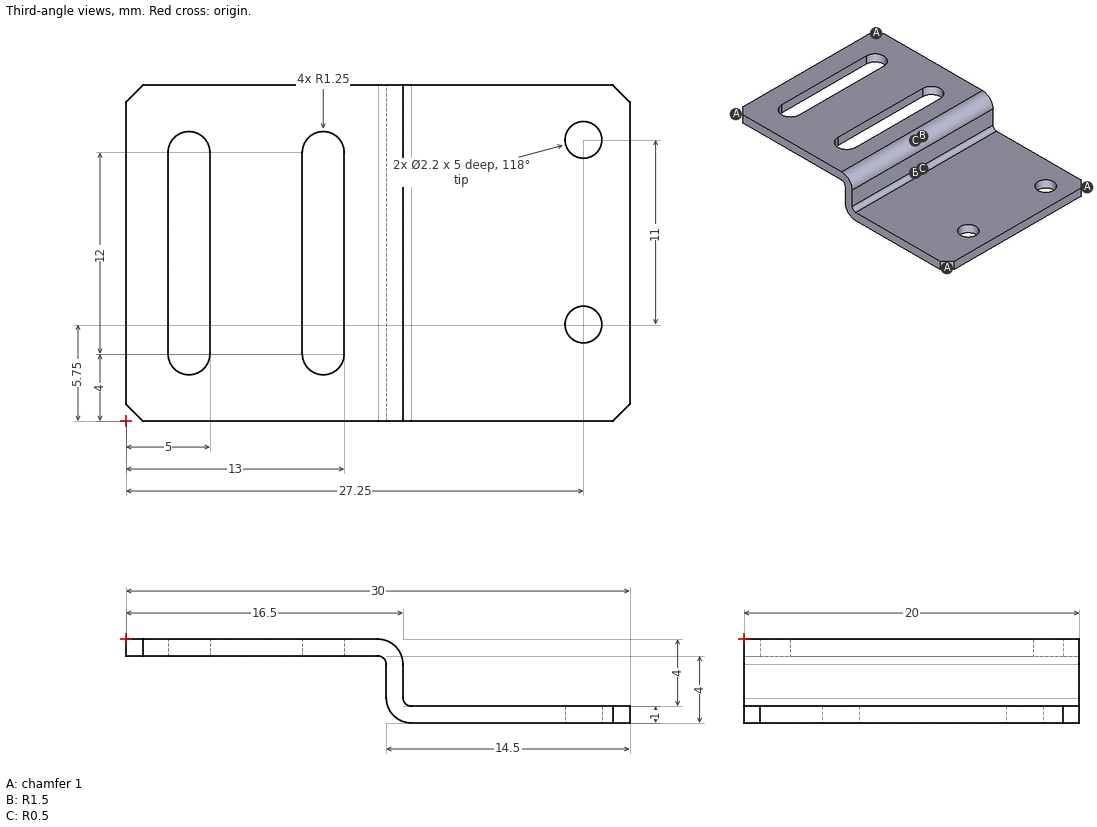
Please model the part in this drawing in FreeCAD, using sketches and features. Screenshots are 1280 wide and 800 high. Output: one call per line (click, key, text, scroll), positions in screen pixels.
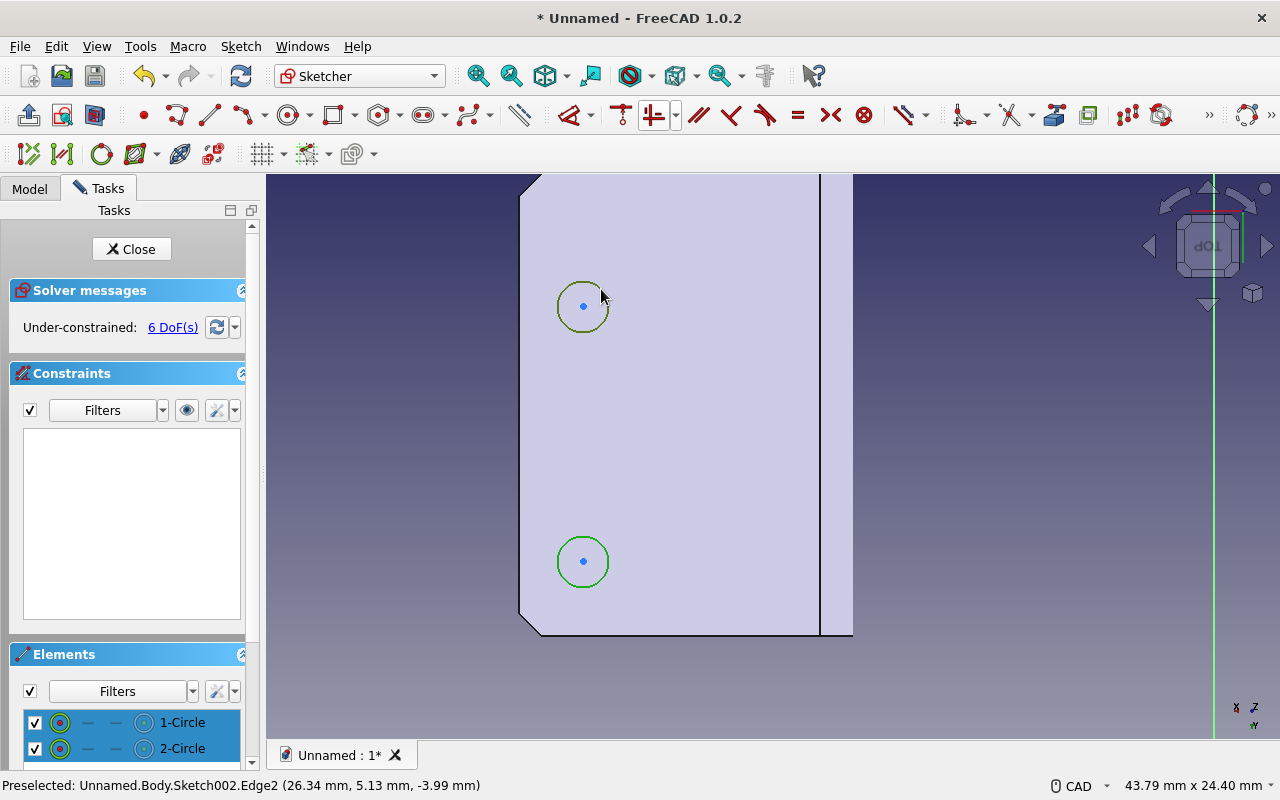
click(798, 116)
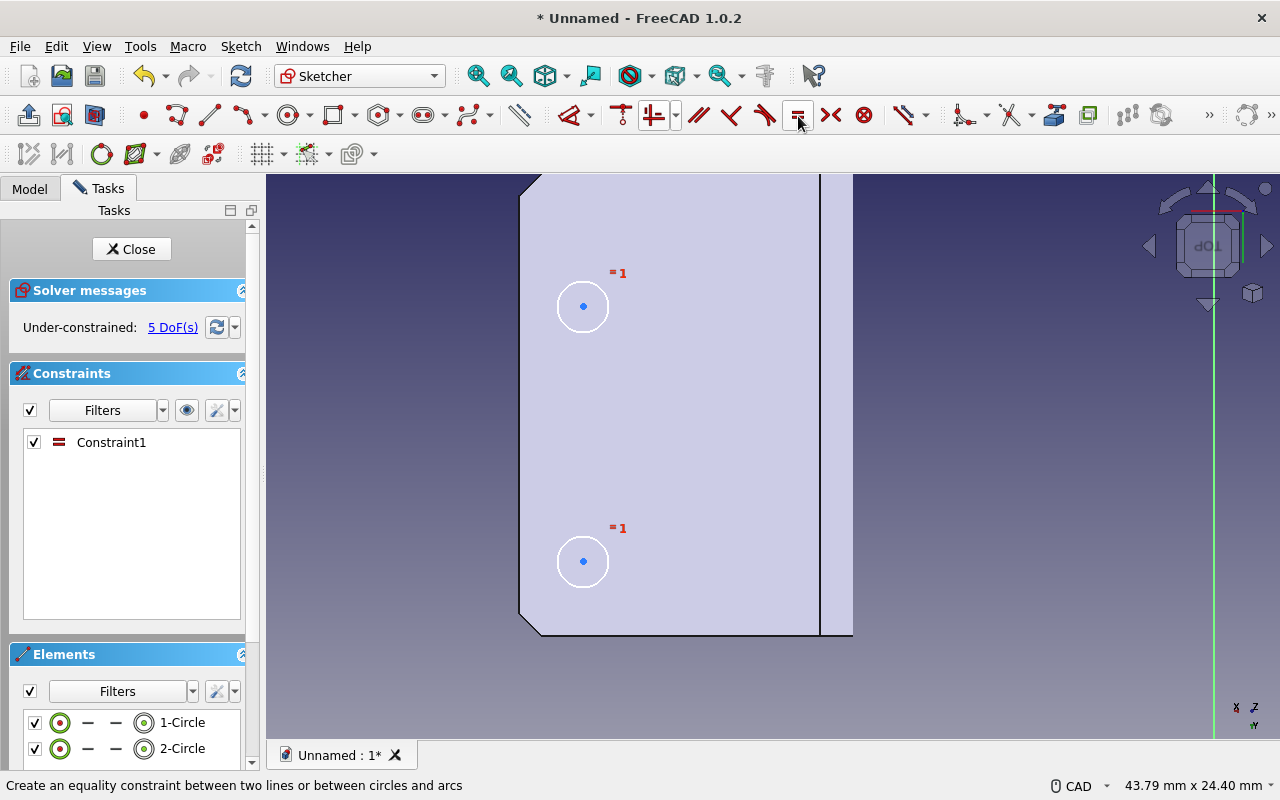
click(583, 562)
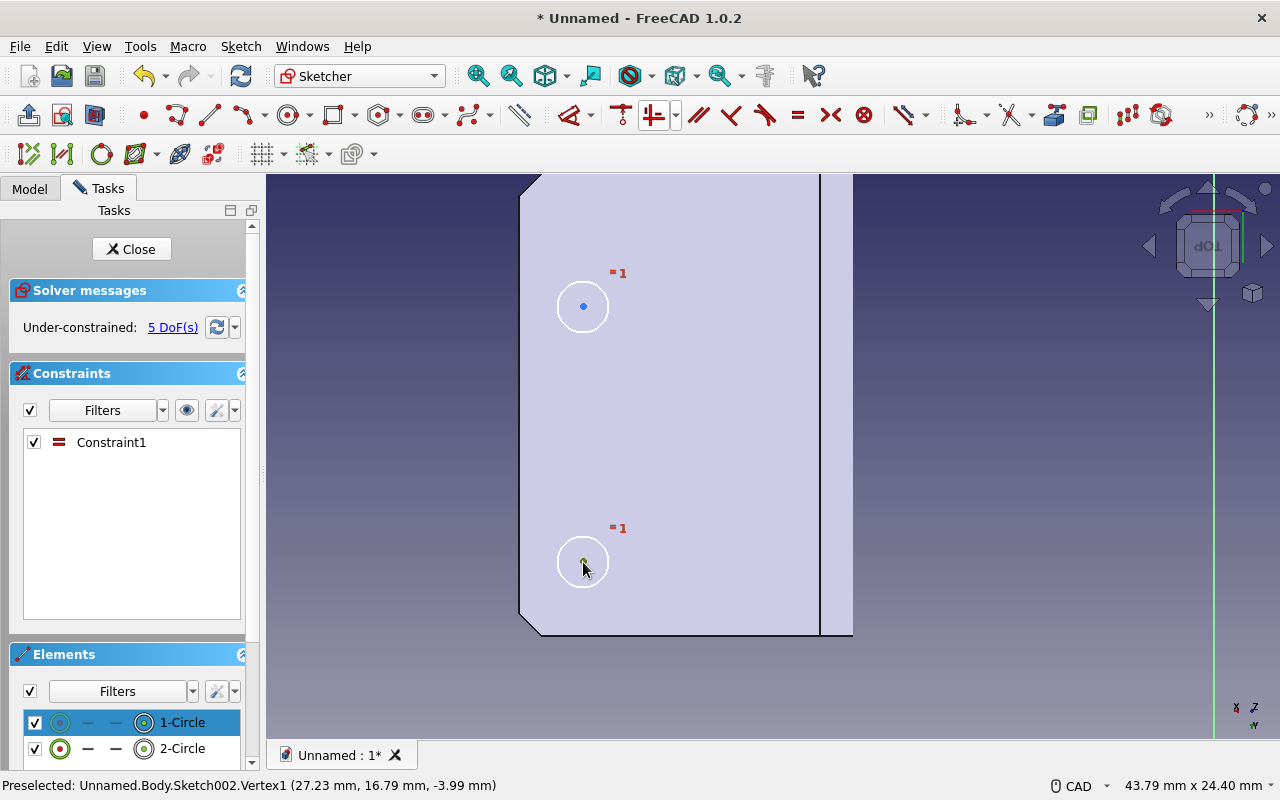
click(583, 307)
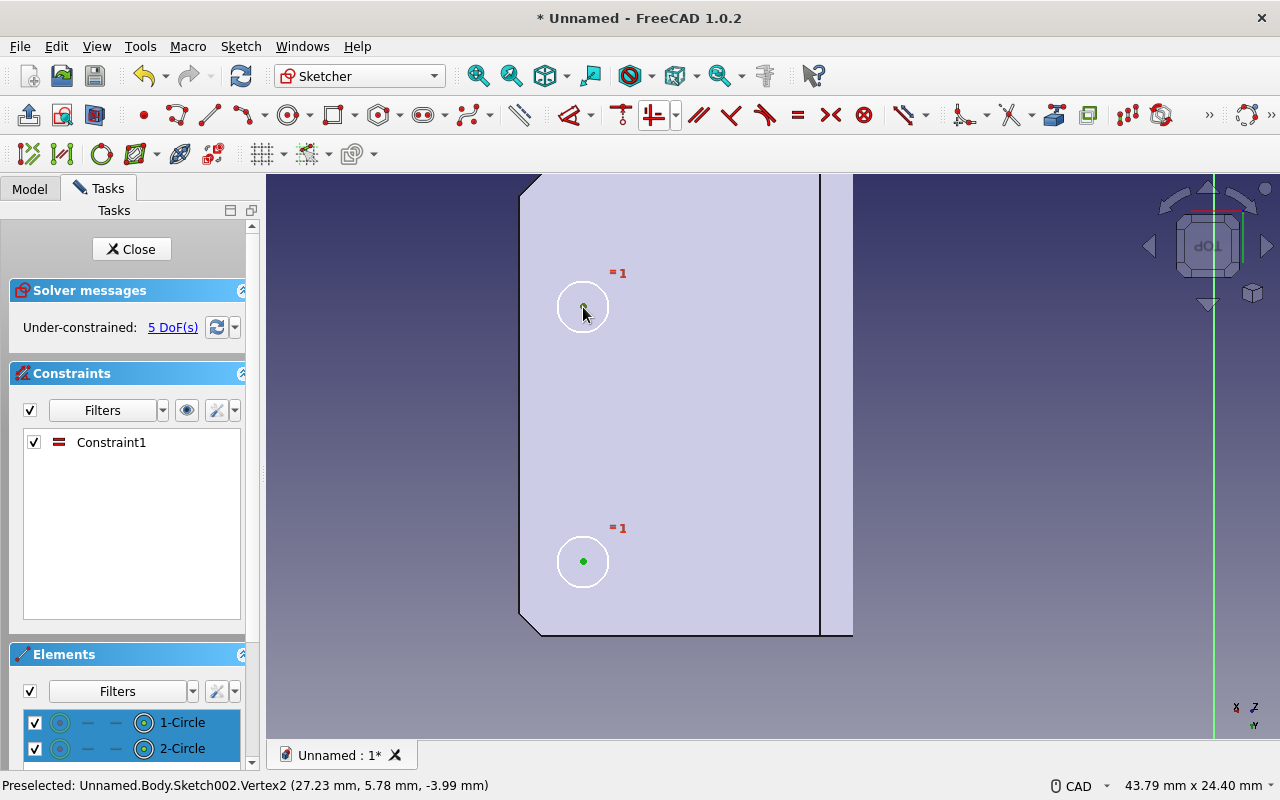
click(676, 116)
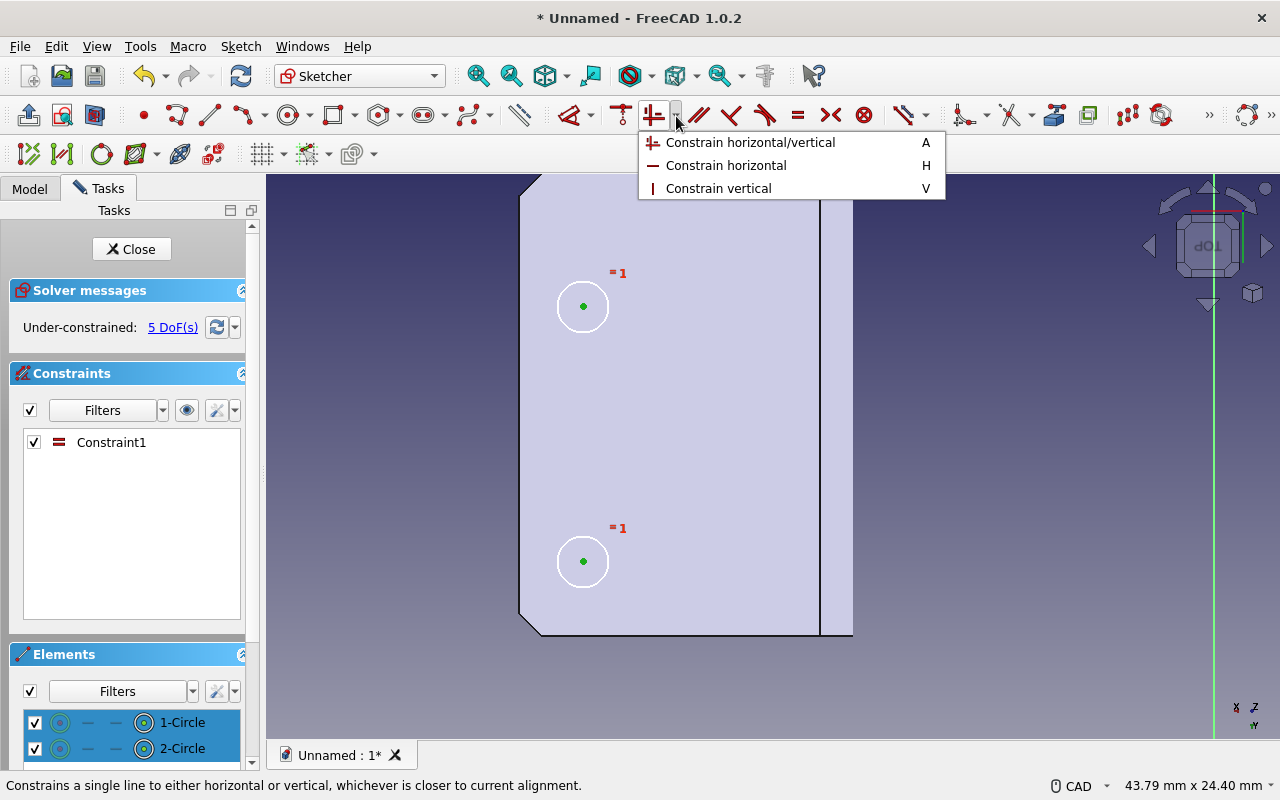
click(792, 188)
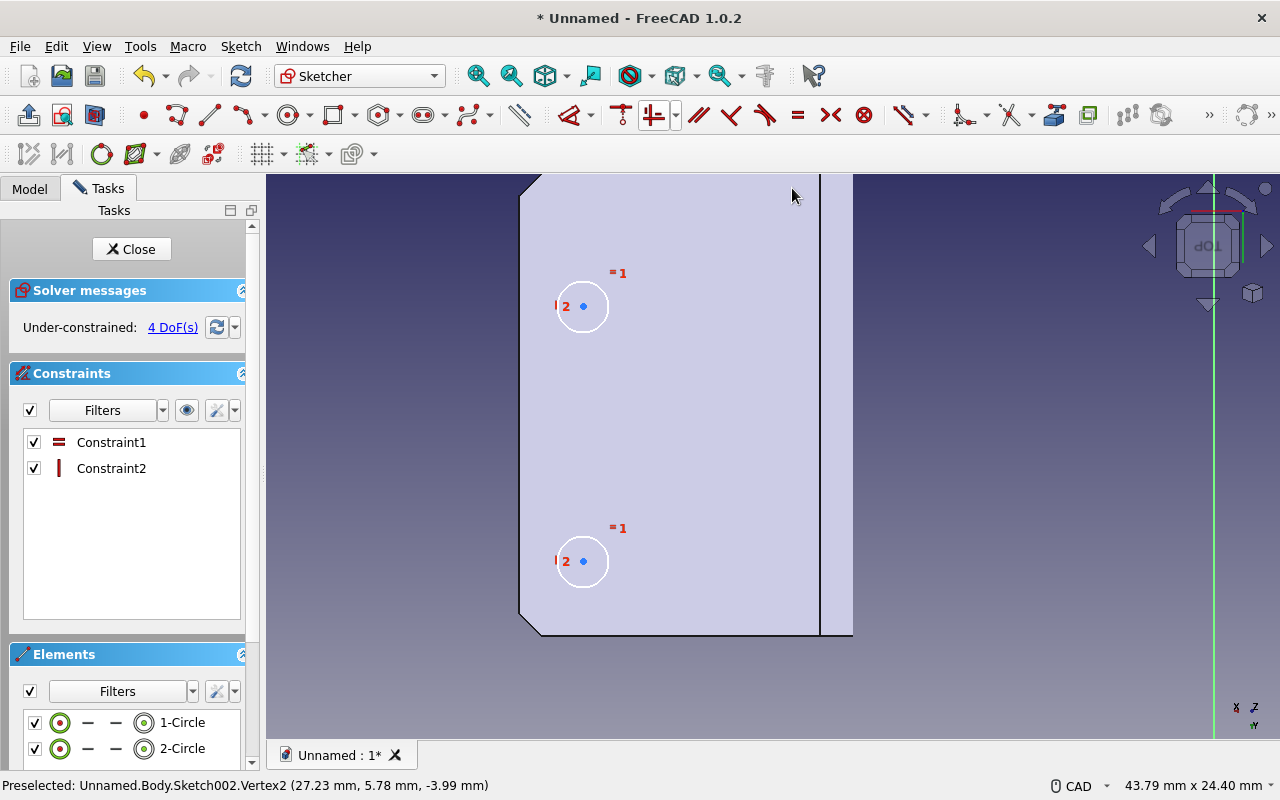
click(568, 116)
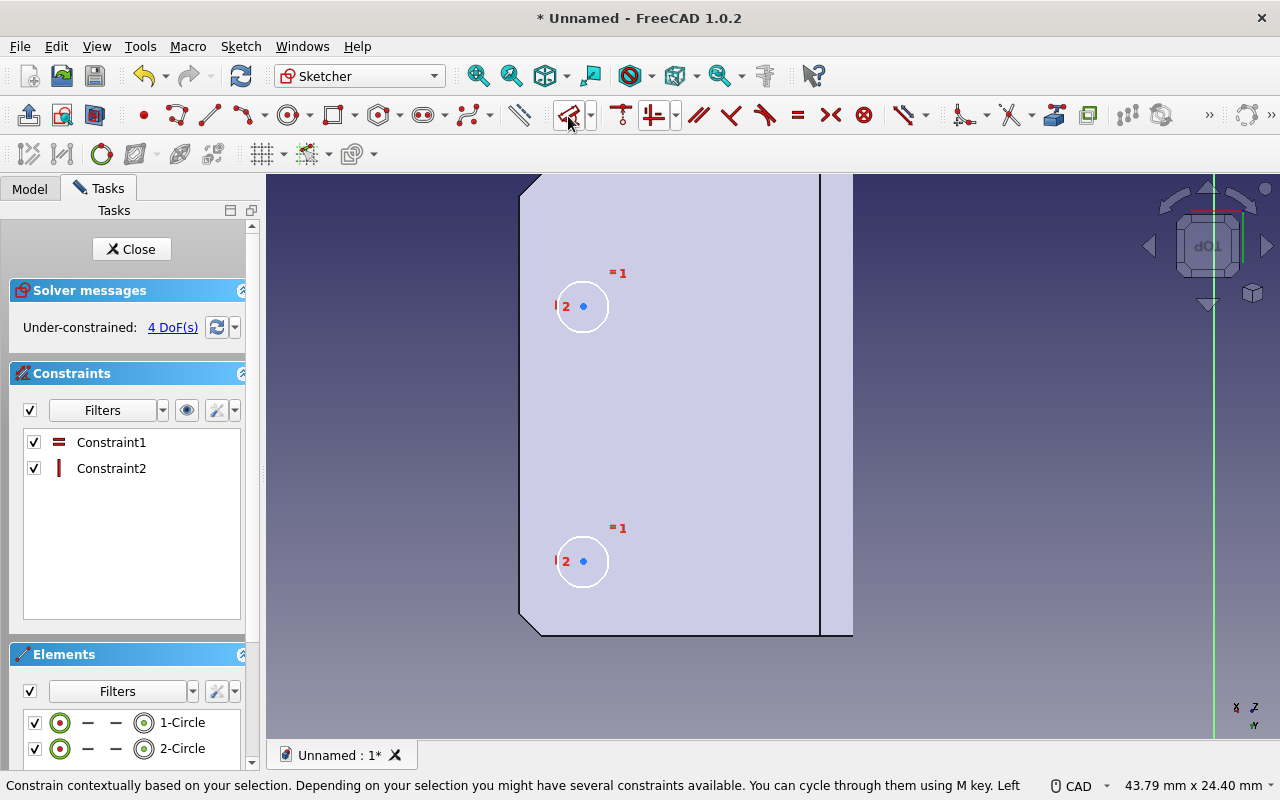
click(601, 544)
click(624, 521)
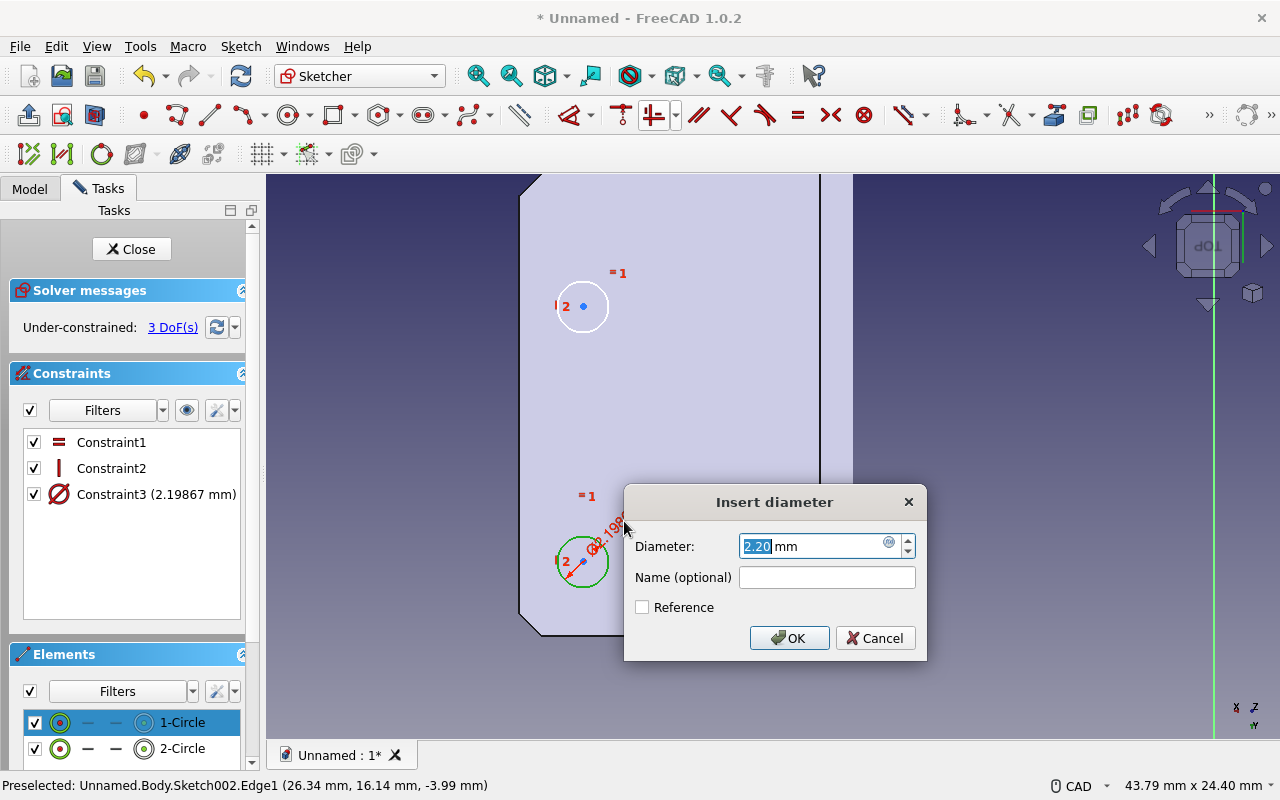
text(2.2)
key(Return)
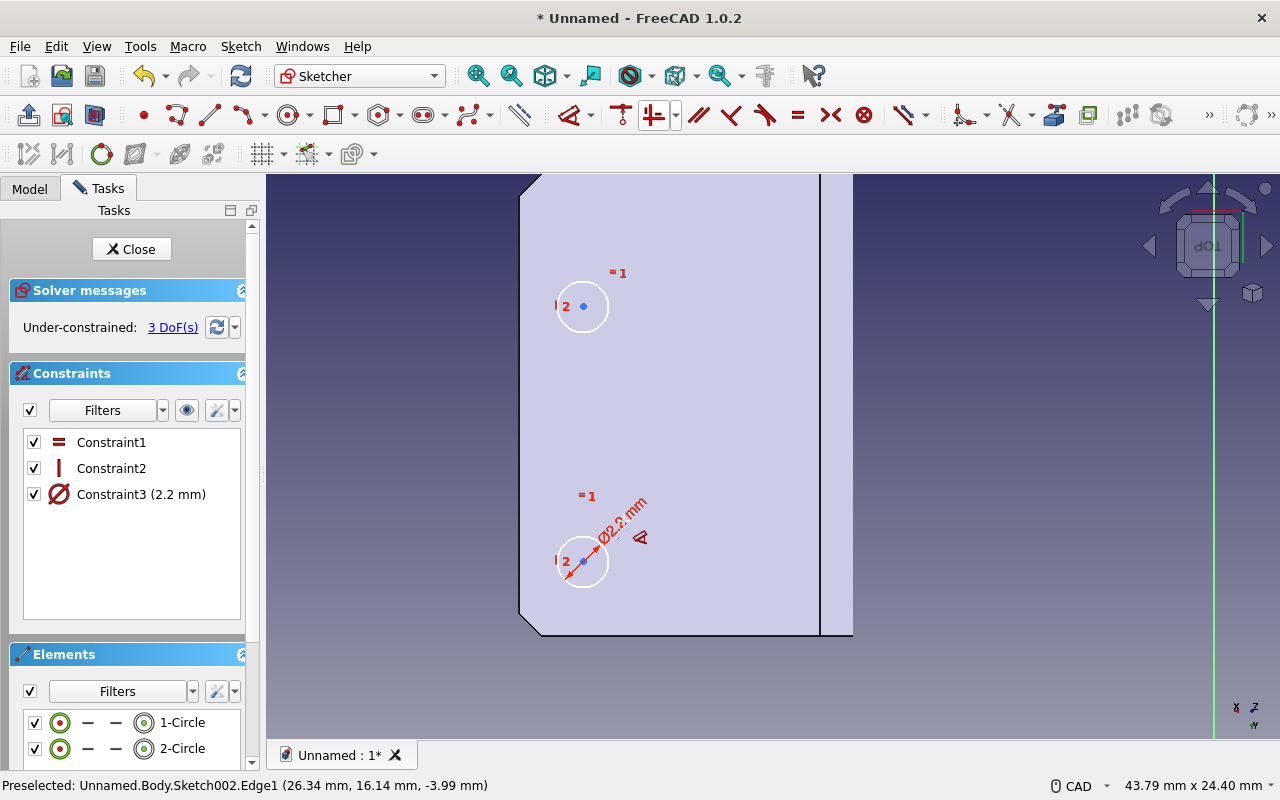
click(583, 562)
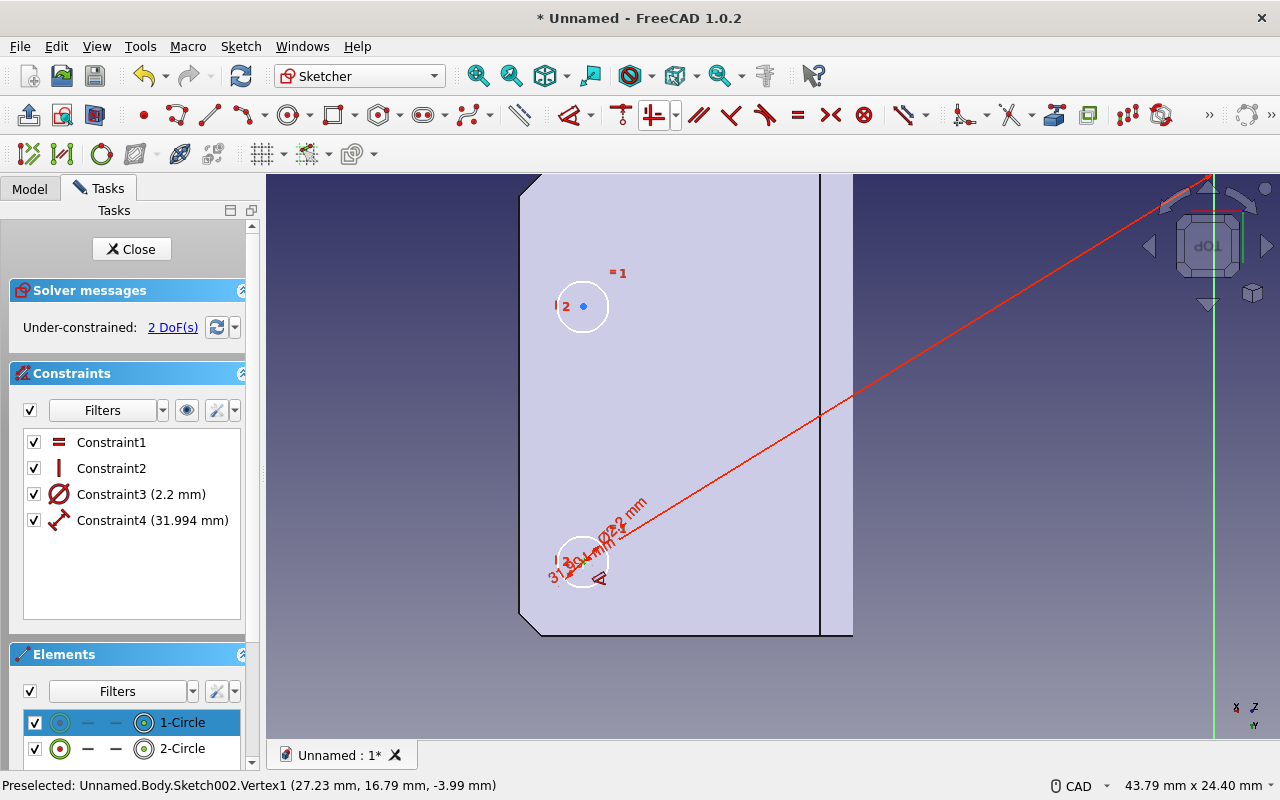
click(583, 307)
click(549, 435)